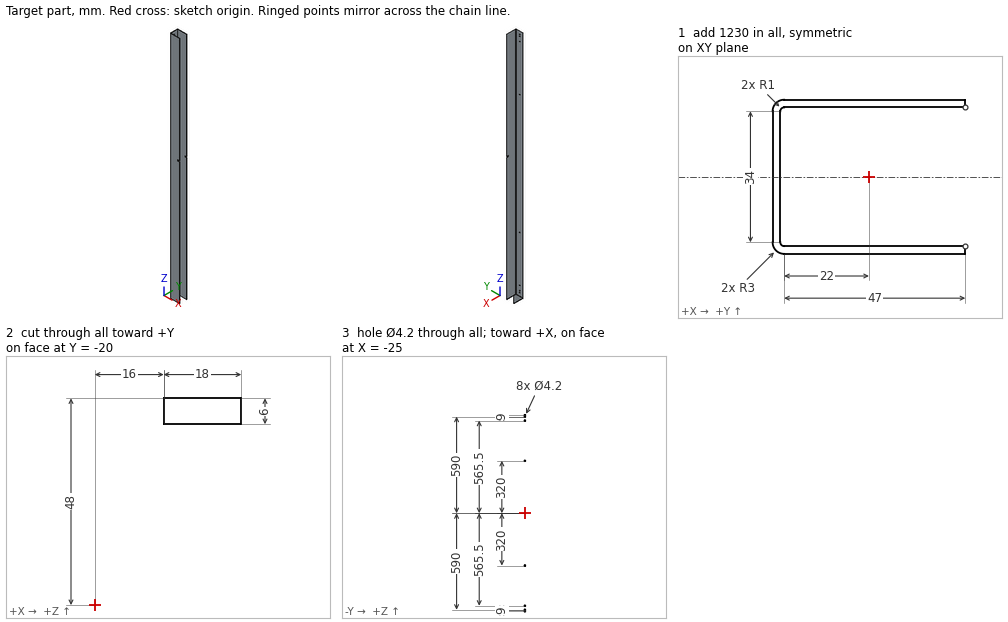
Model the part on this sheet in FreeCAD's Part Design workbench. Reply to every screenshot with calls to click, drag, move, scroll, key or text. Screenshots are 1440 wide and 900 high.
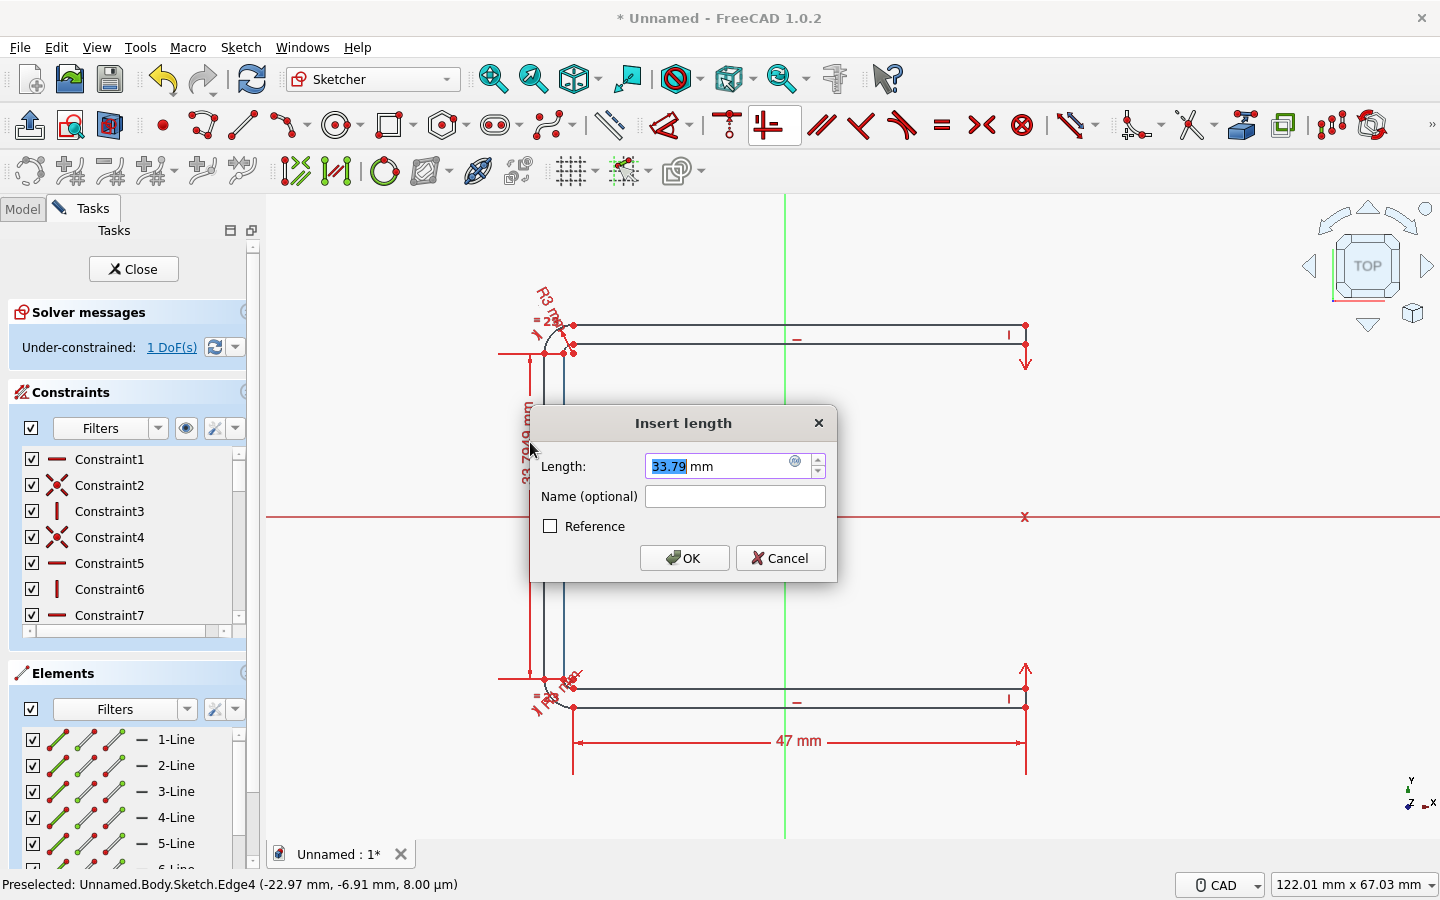
text(34)
key(Return)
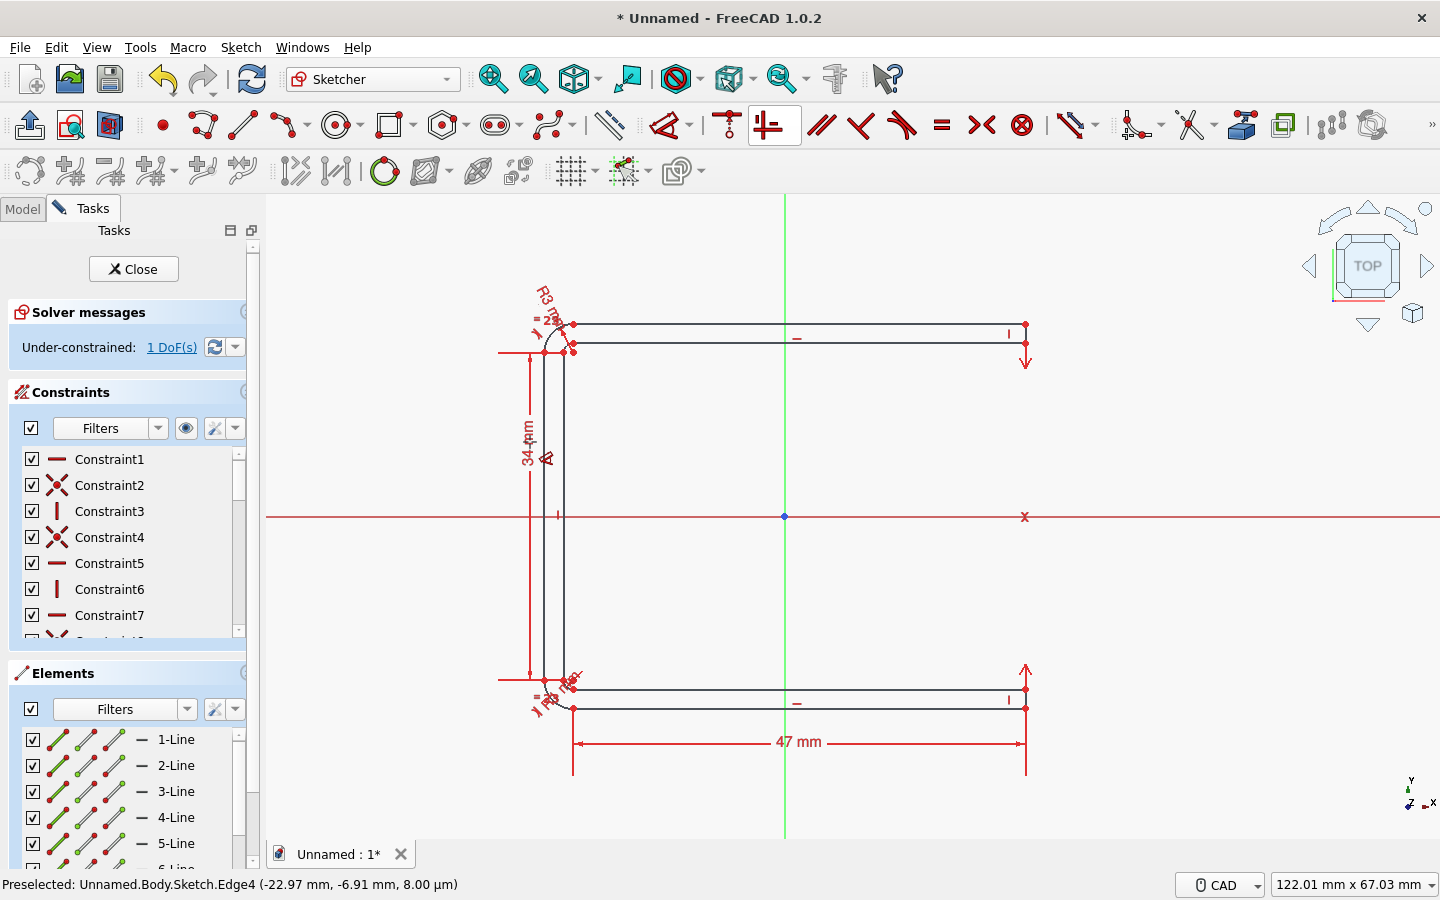
click(573, 709)
click(679, 743)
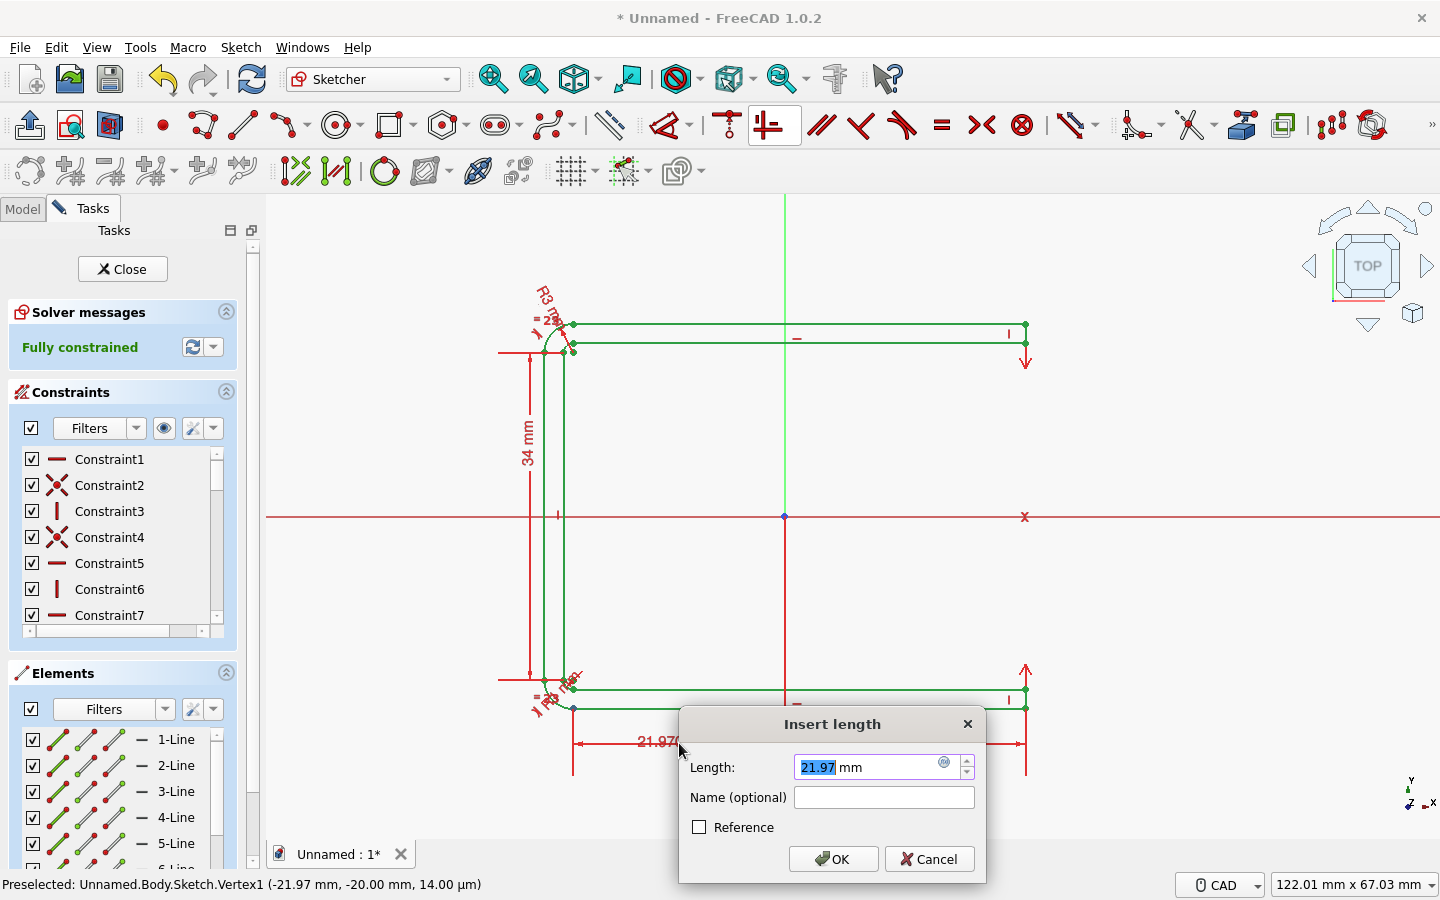
text(22)
key(Return)
key(Escape)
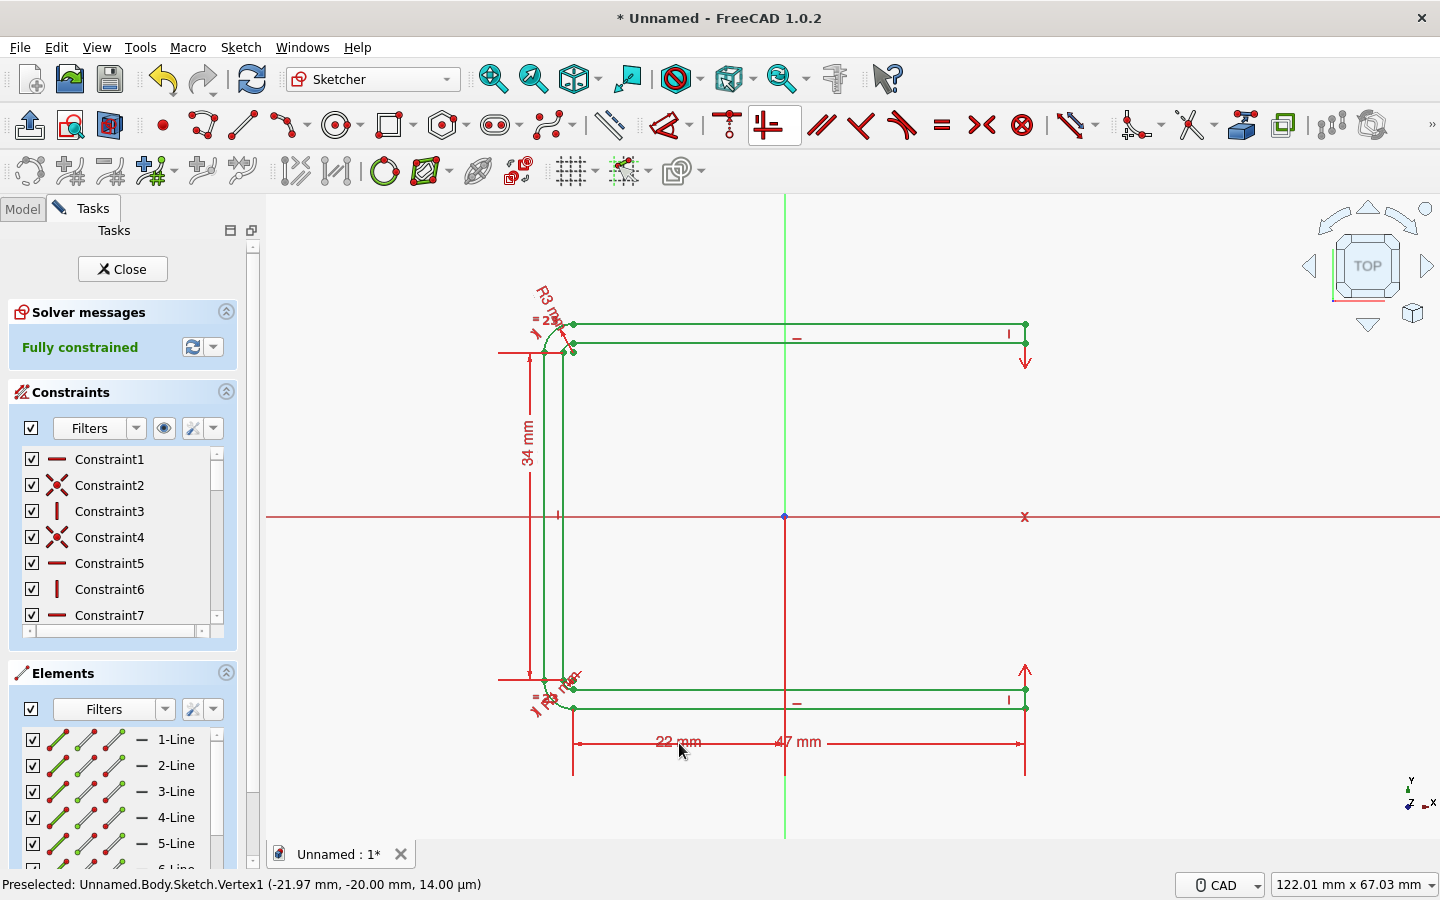
click(123, 269)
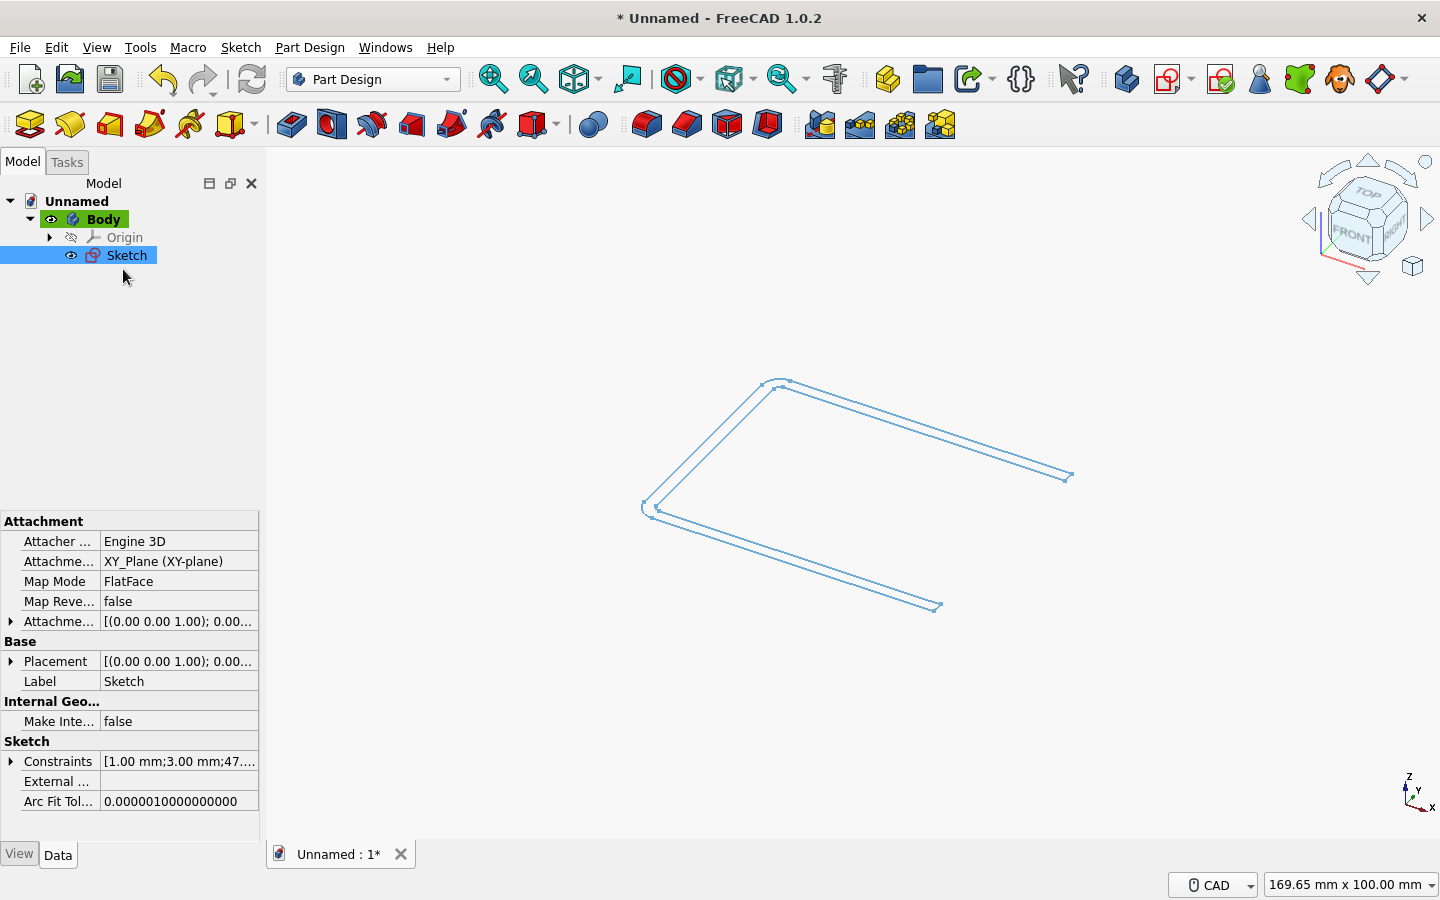
click(30, 124)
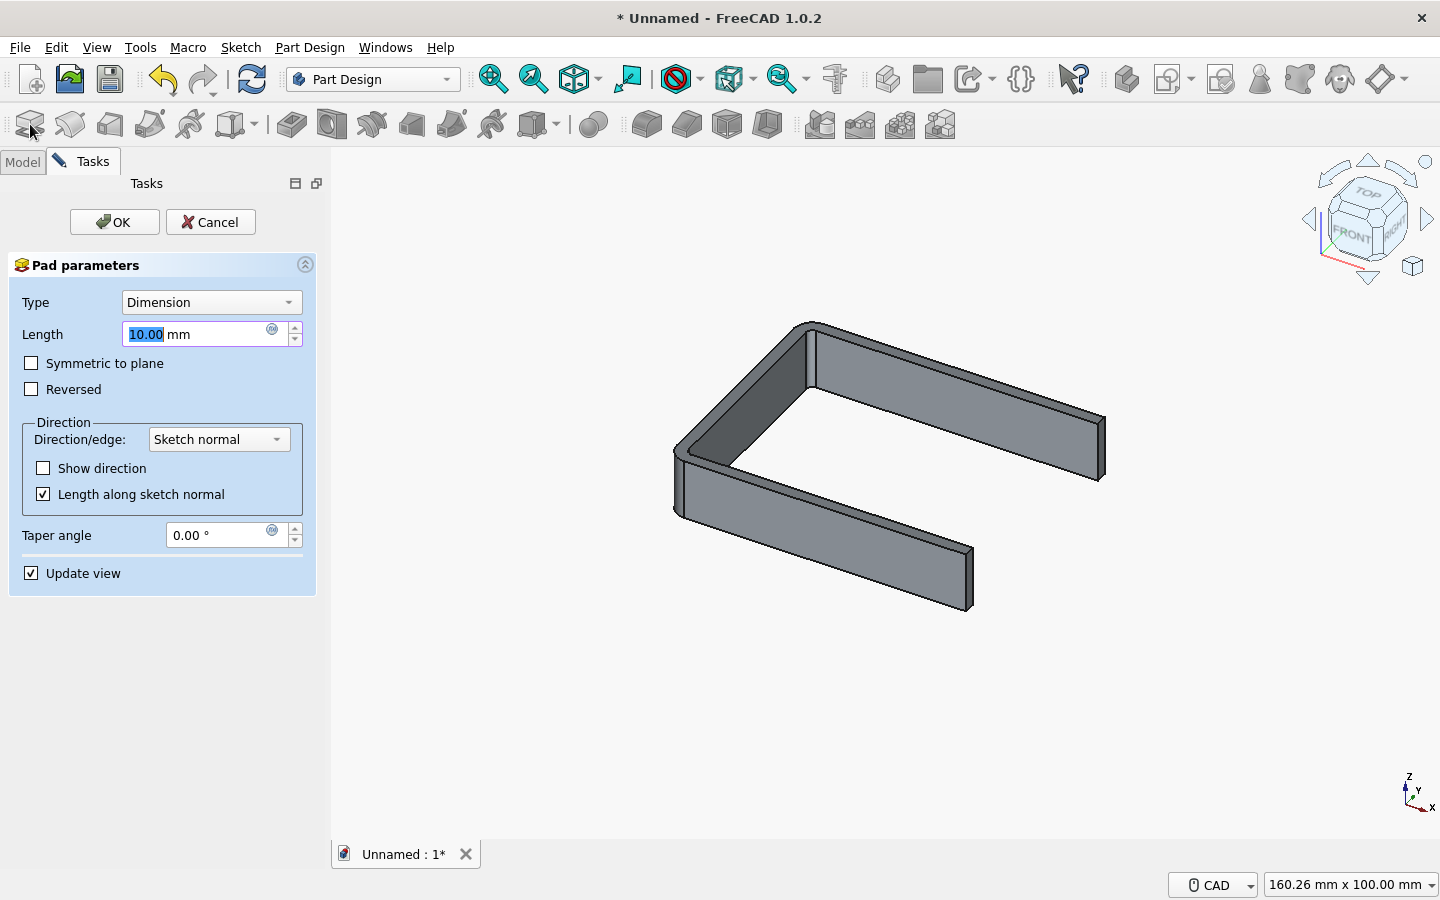
text(1230)
key(Tab)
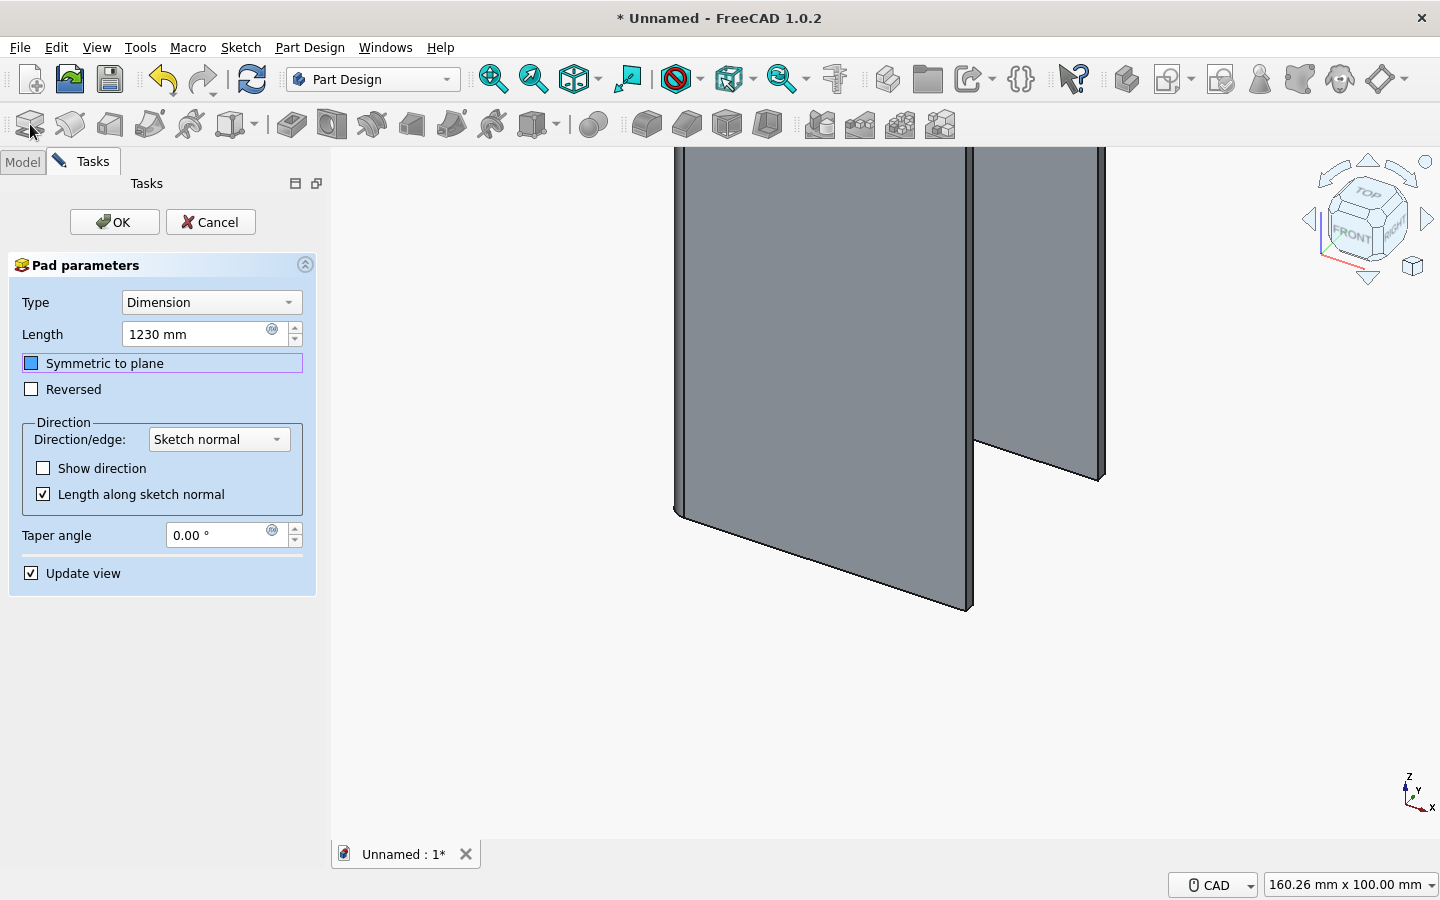
click(30, 363)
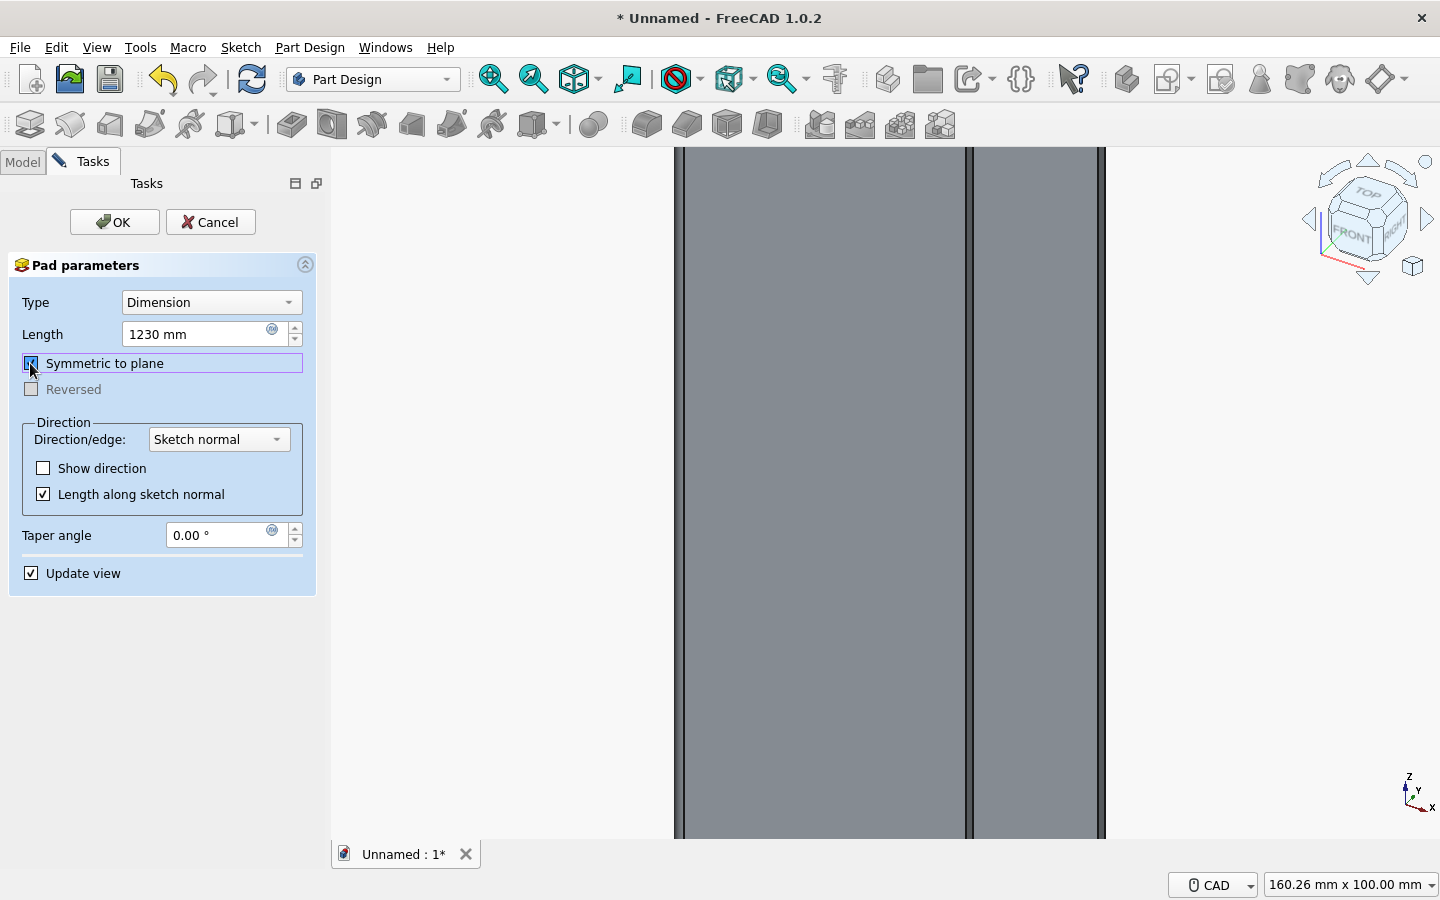
click(115, 222)